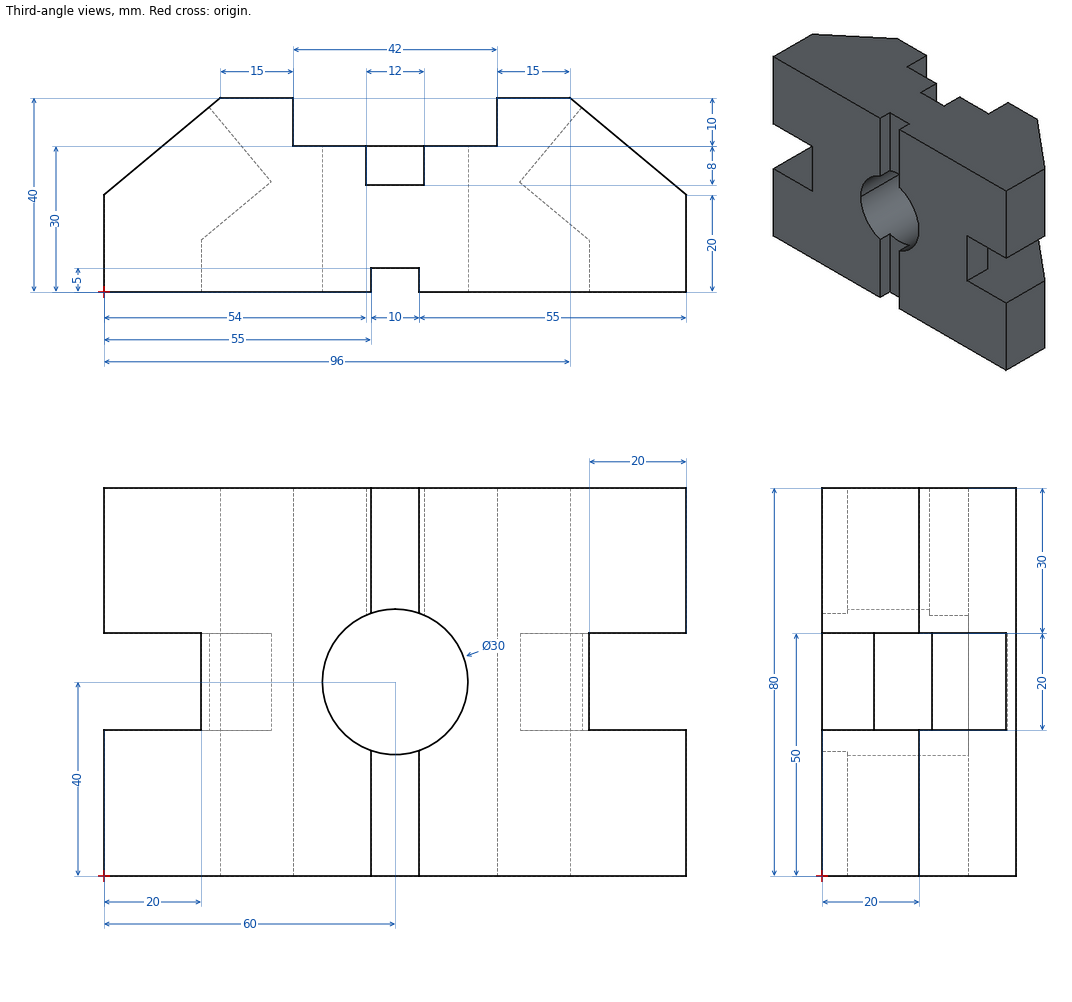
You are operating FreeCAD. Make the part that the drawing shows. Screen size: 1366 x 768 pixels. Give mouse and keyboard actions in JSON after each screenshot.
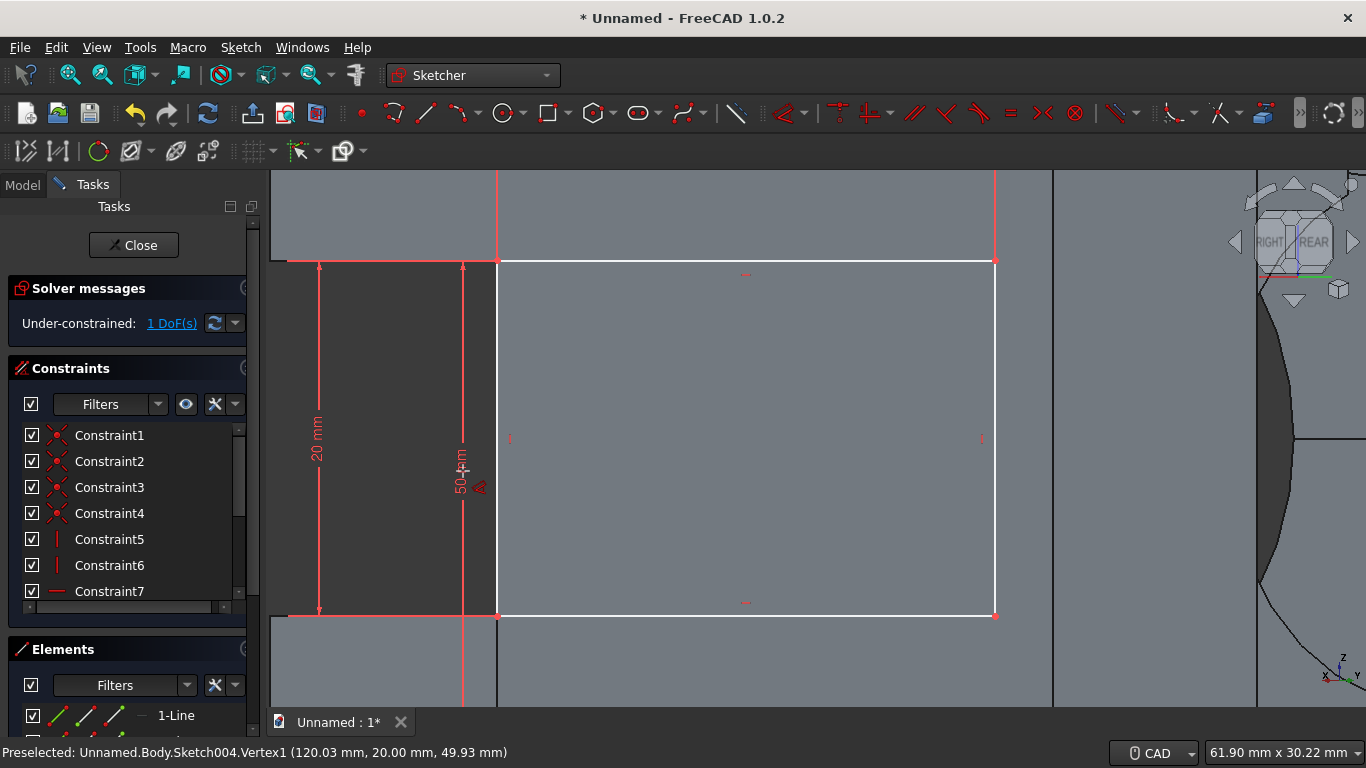
{"action": "left_click", "coordinate": [497, 261]}
{"action": "left_click", "coordinate": [849, 227]}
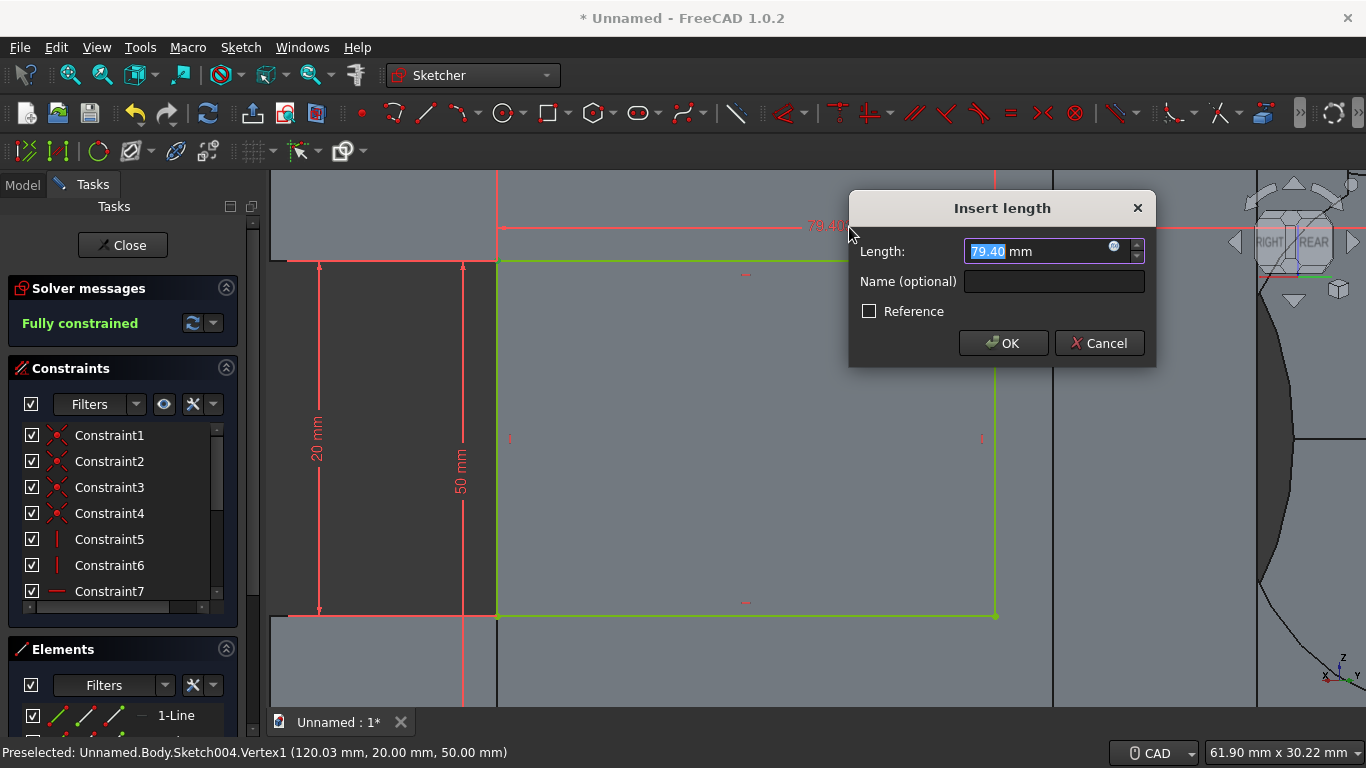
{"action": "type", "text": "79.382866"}
{"action": "key", "text": "Return"}
{"action": "key", "text": "Escape"}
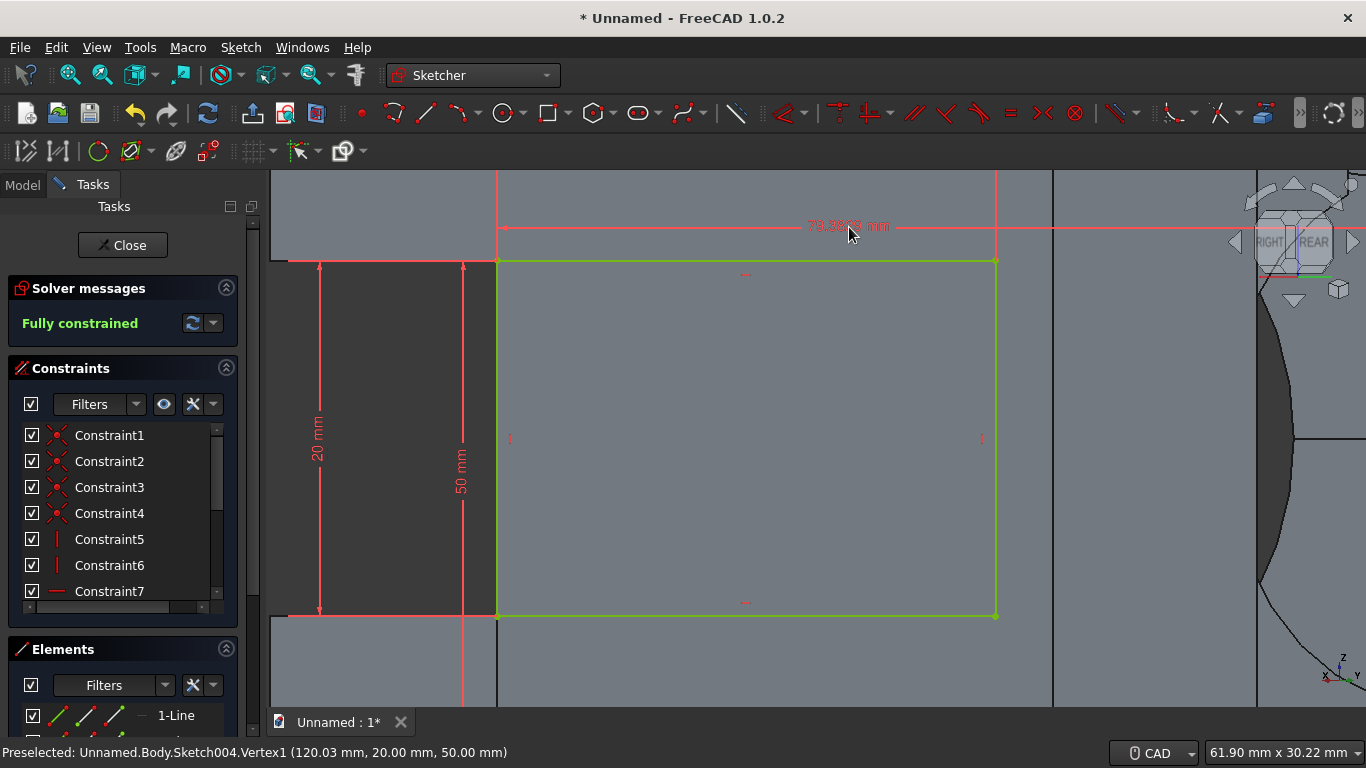
{"action": "left_click", "coordinate": [123, 245]}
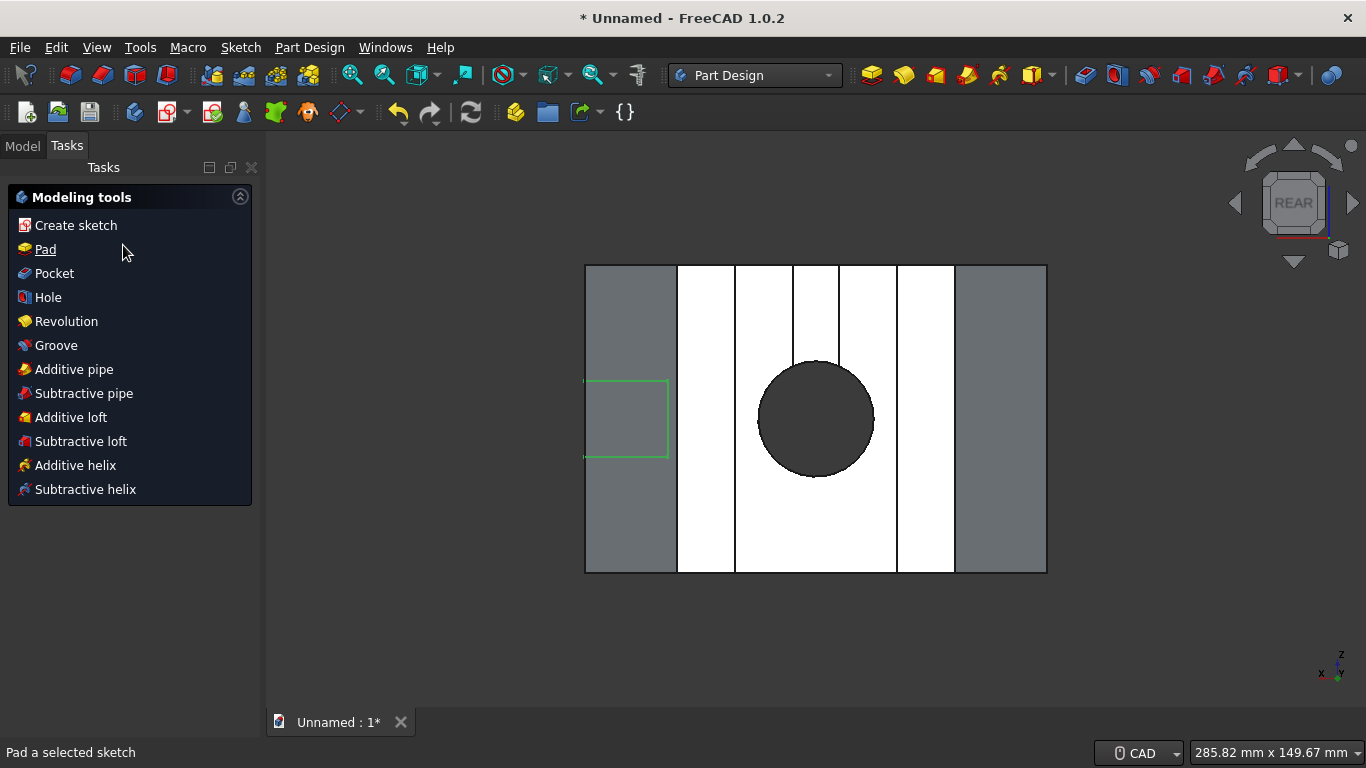
{"action": "left_click", "coordinate": [1086, 76]}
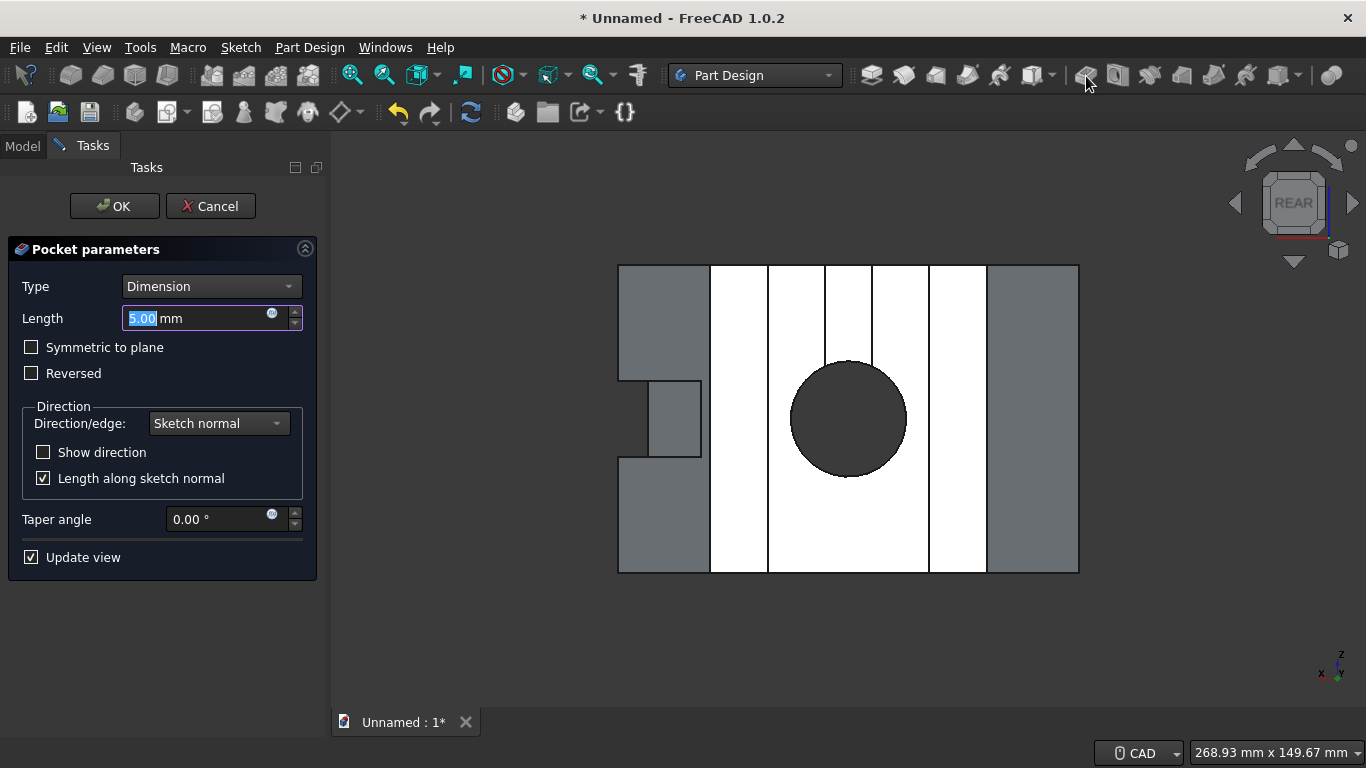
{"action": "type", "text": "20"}
{"action": "key", "text": "Tab"}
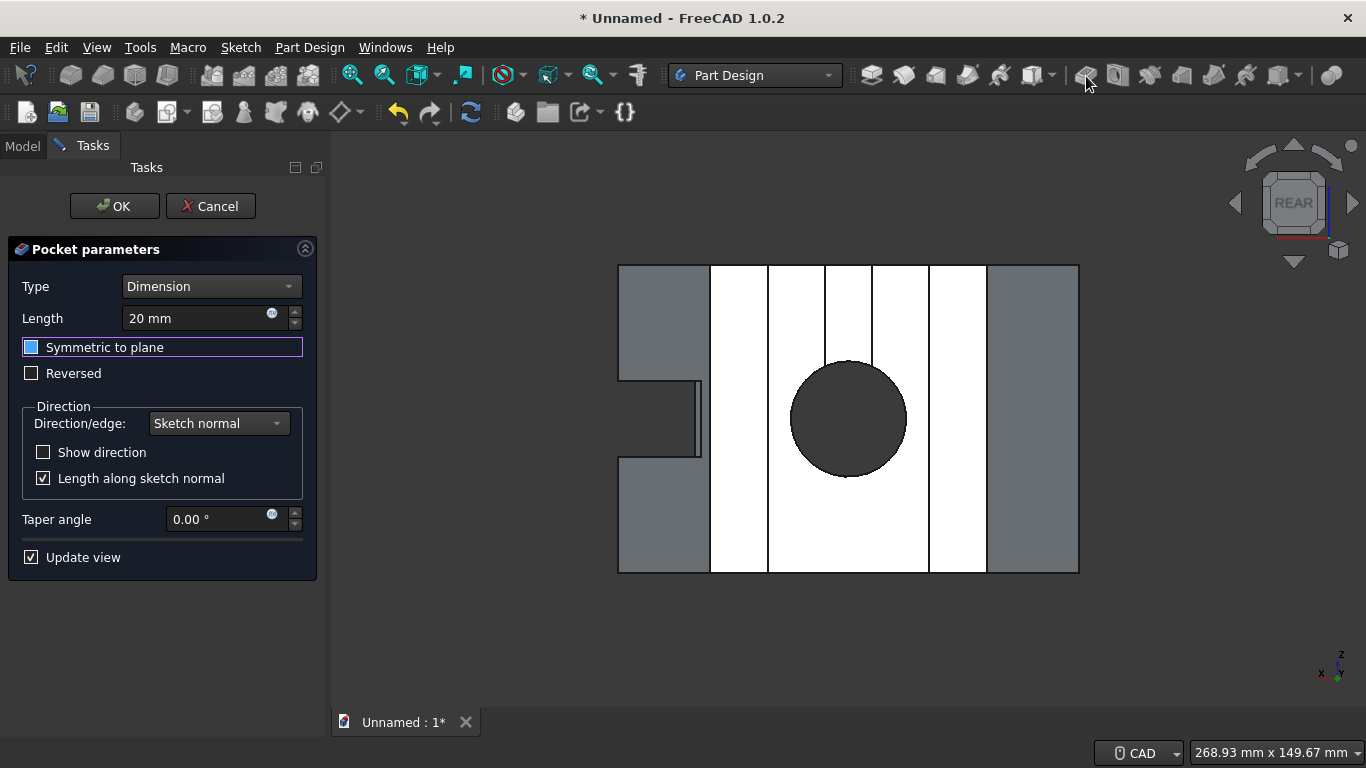
{"action": "left_click", "coordinate": [115, 206]}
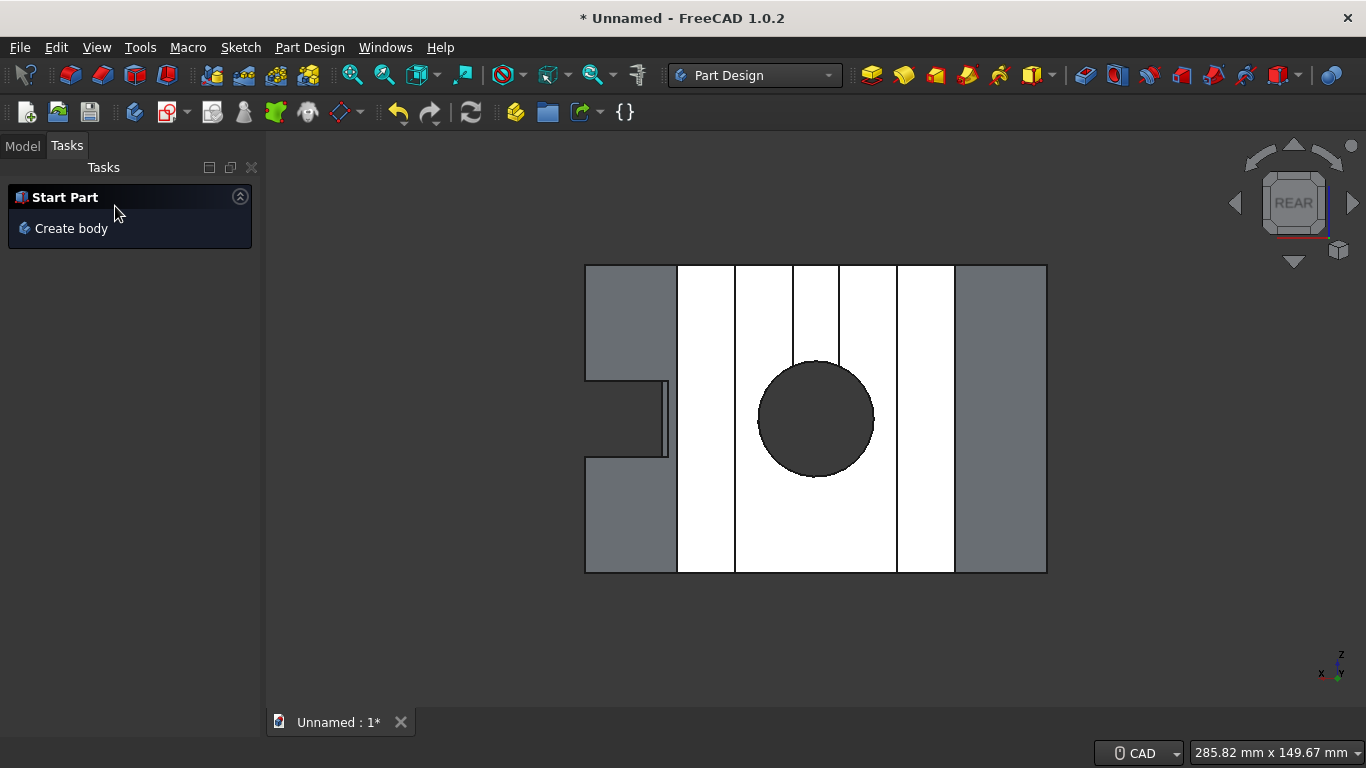
{"action": "key", "text": "6"}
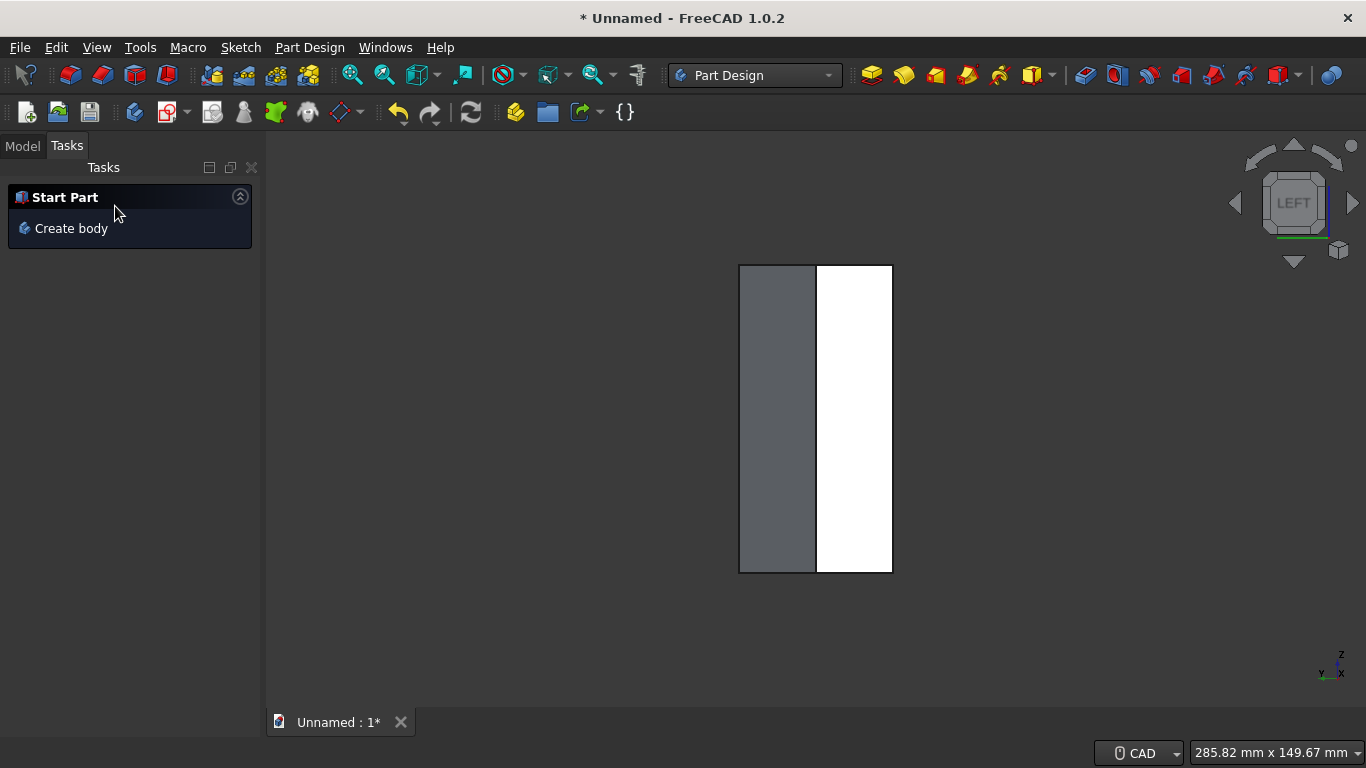
{"action": "left_click", "coordinate": [854, 330]}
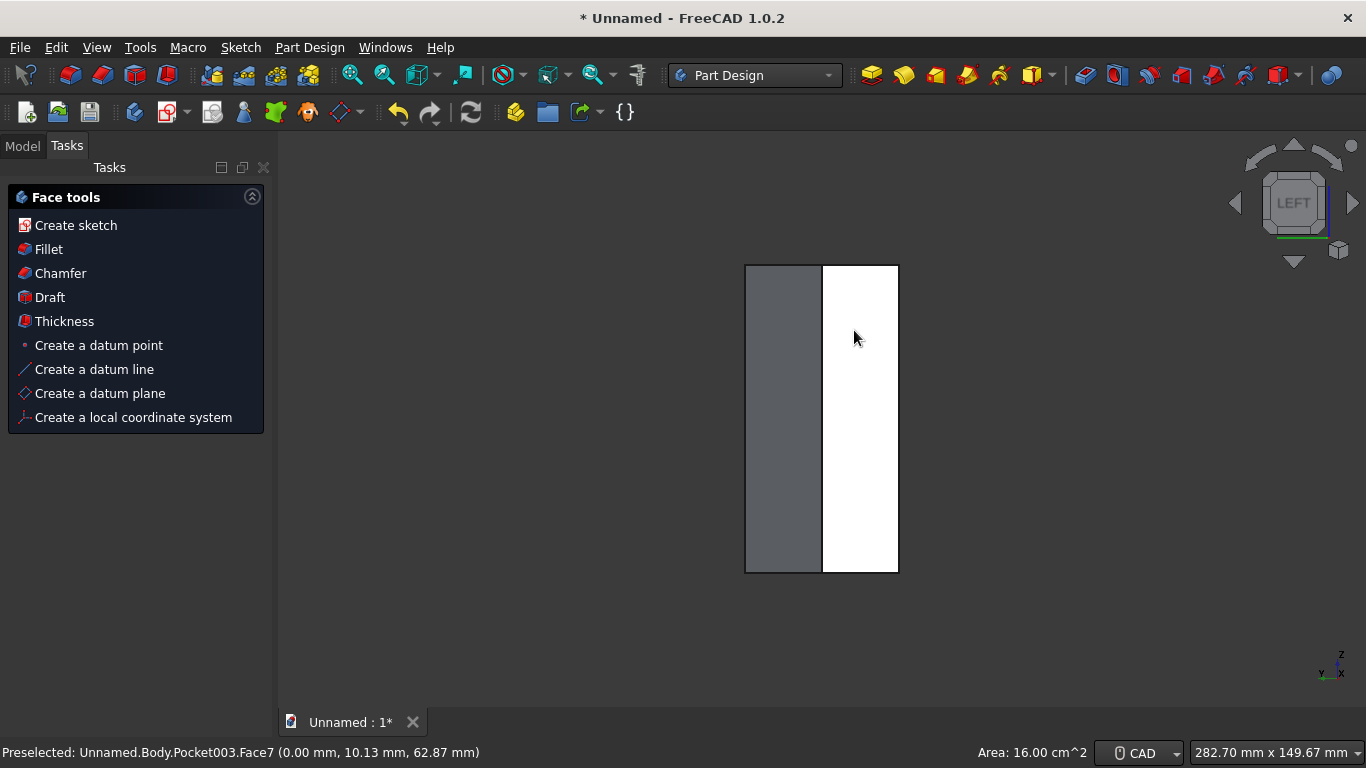
{"action": "left_click", "coordinate": [168, 112]}